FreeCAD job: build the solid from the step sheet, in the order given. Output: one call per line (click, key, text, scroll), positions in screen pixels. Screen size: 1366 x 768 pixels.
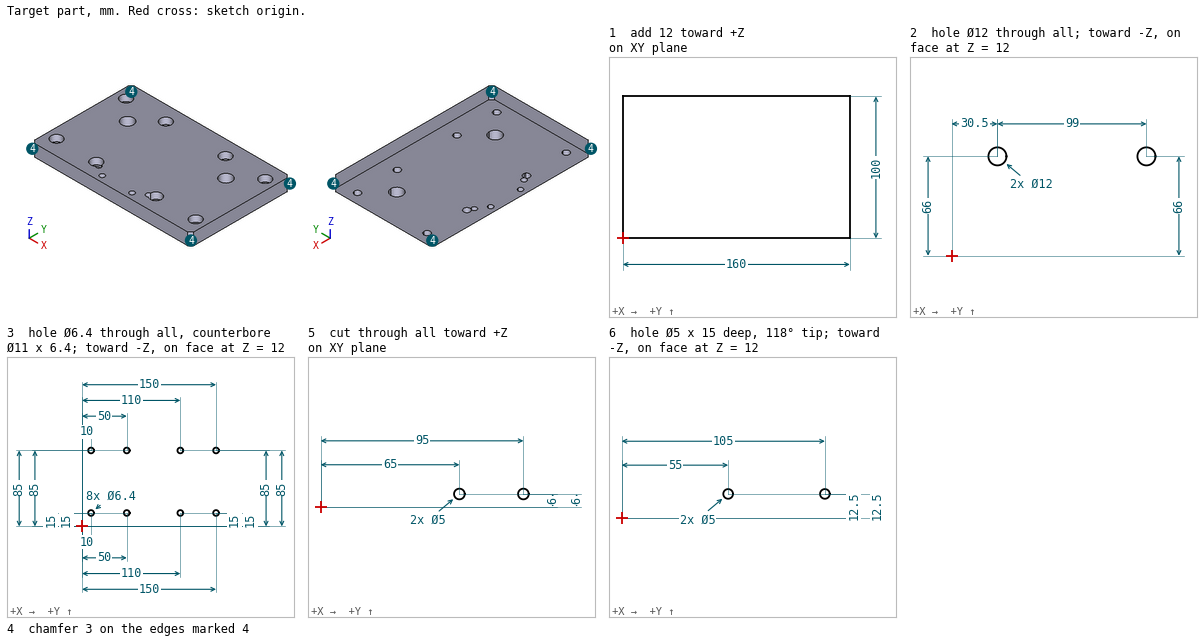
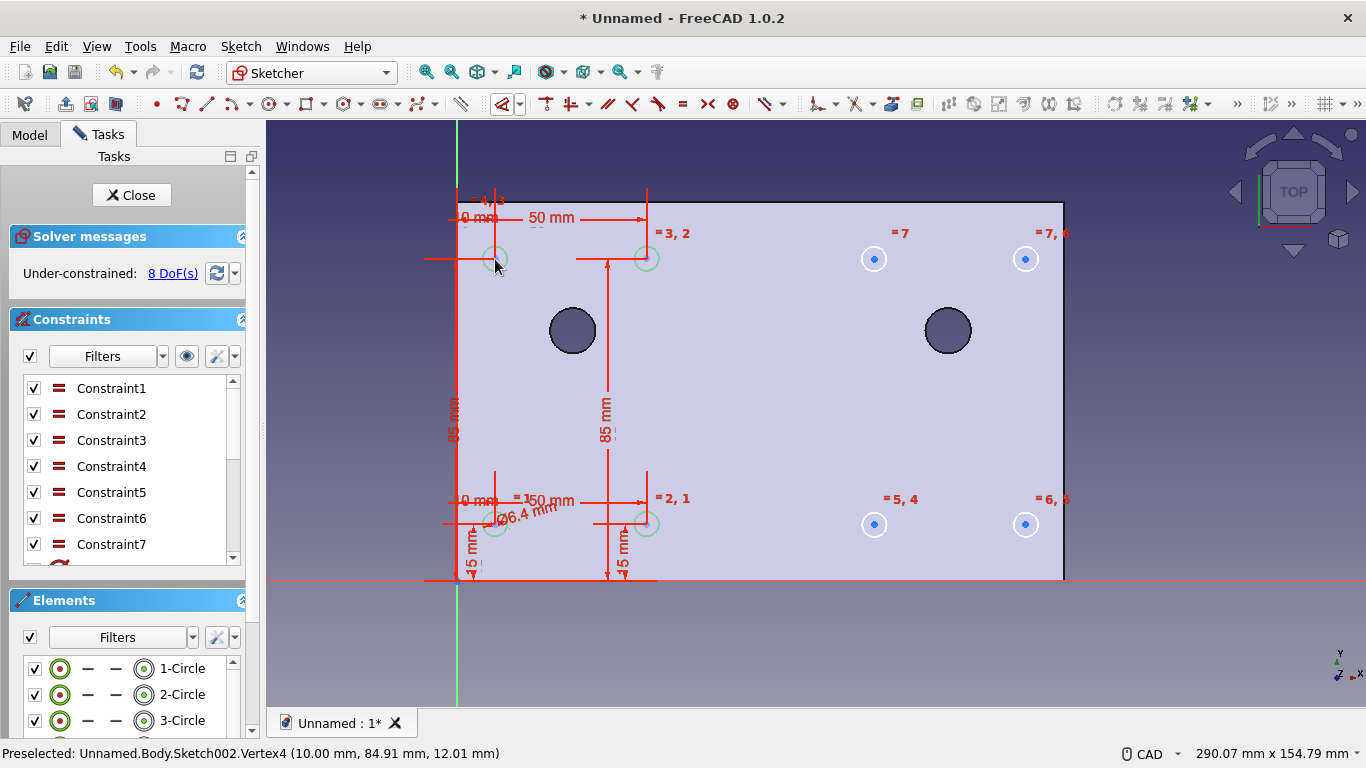
click(874, 525)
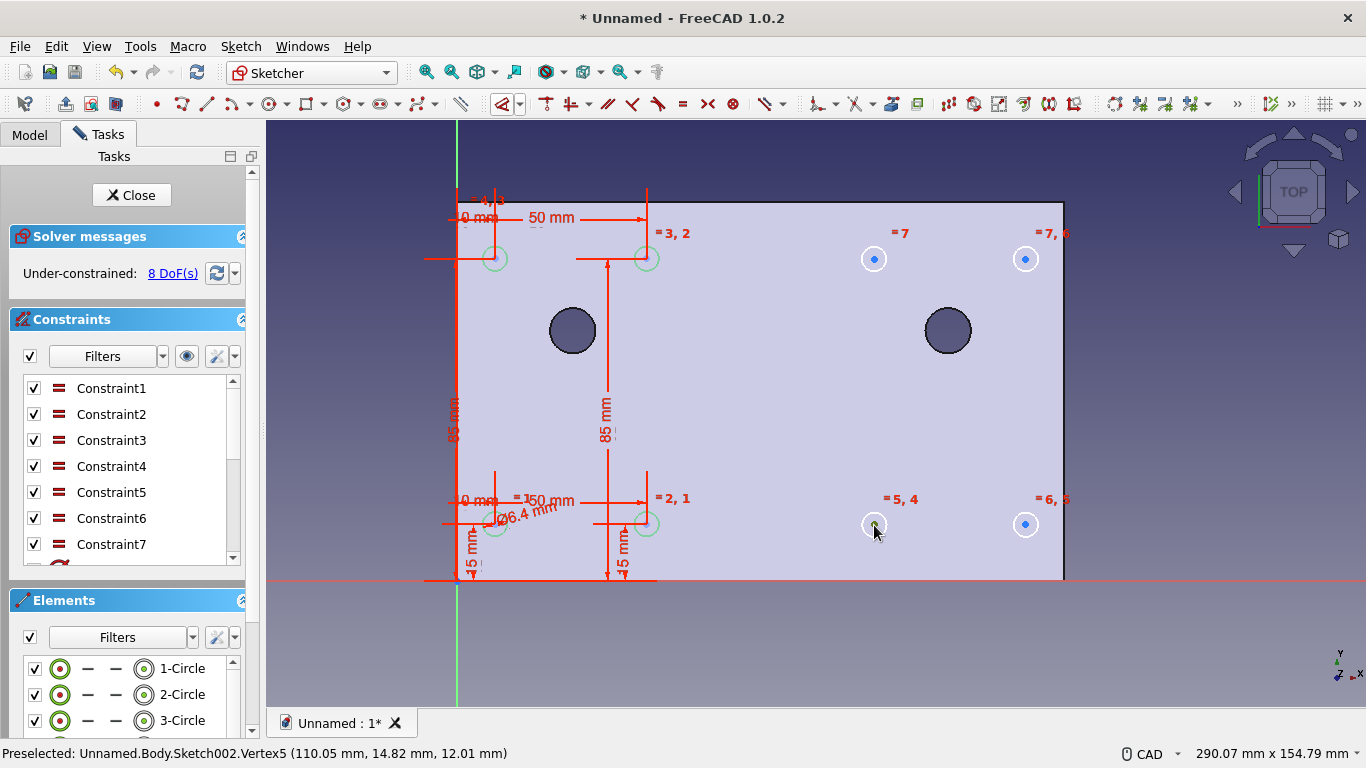
click(520, 104)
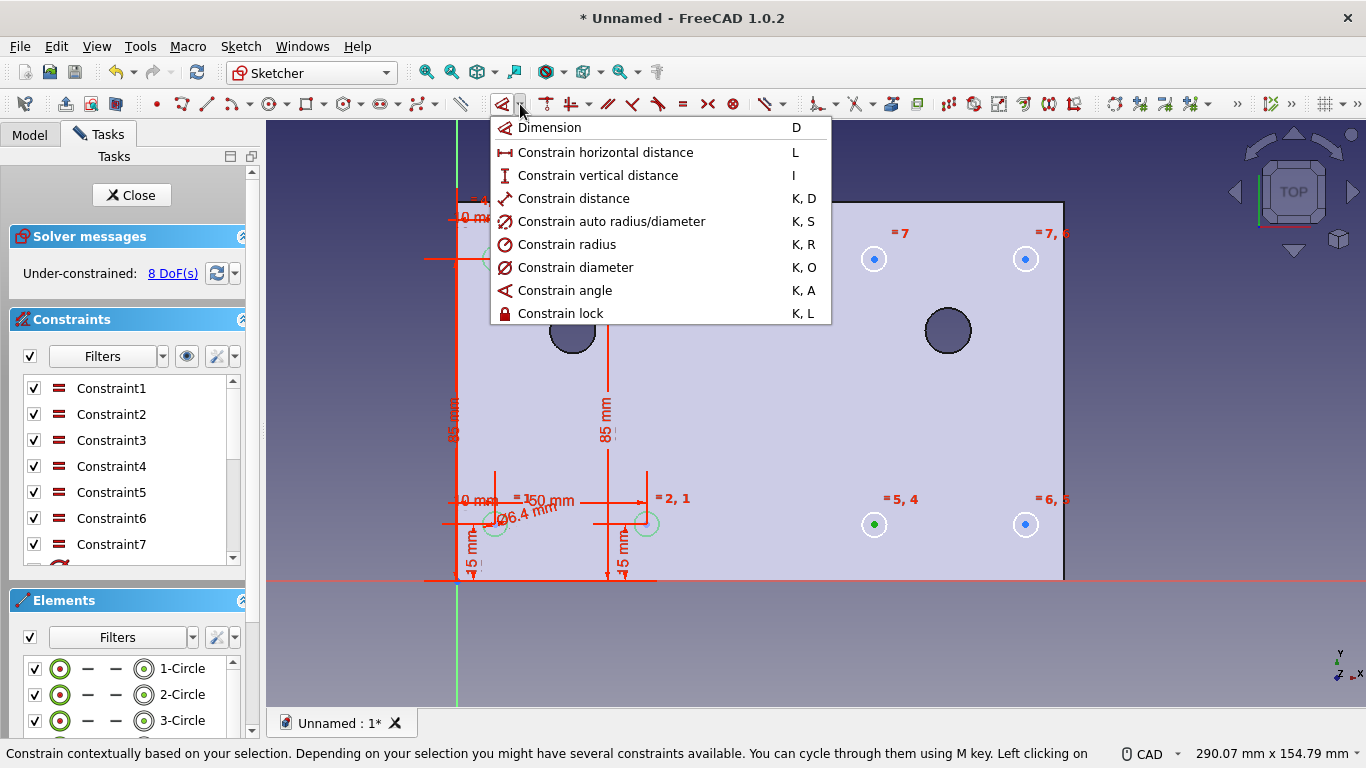
click(661, 176)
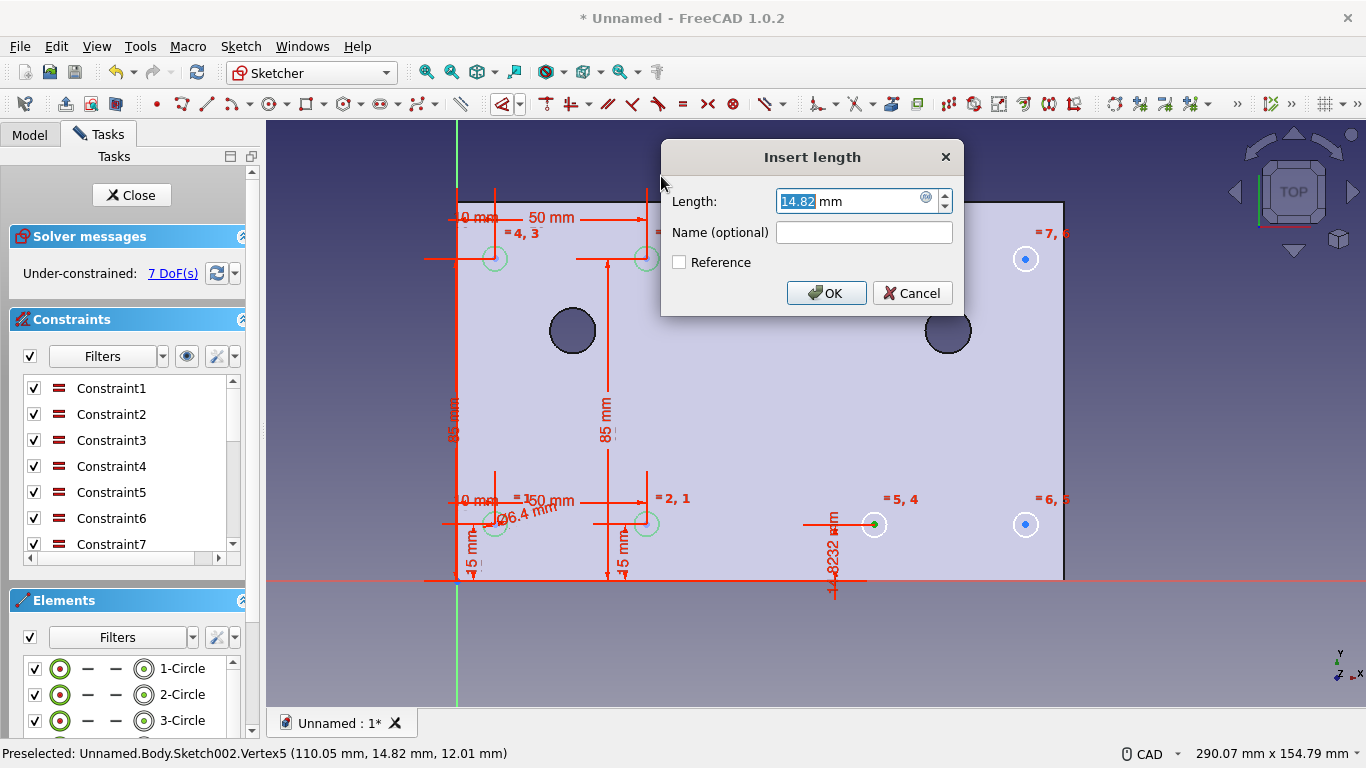
text(15)
key(Return)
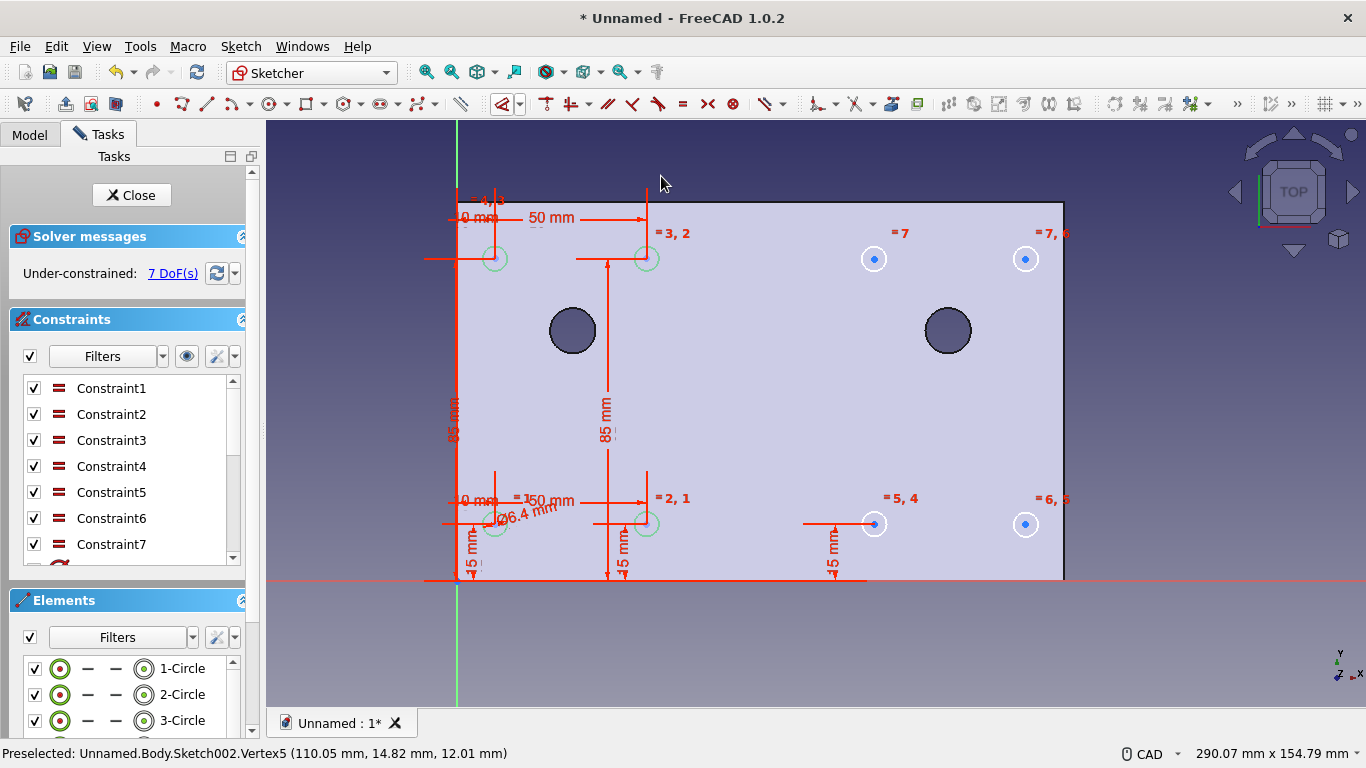
click(1026, 525)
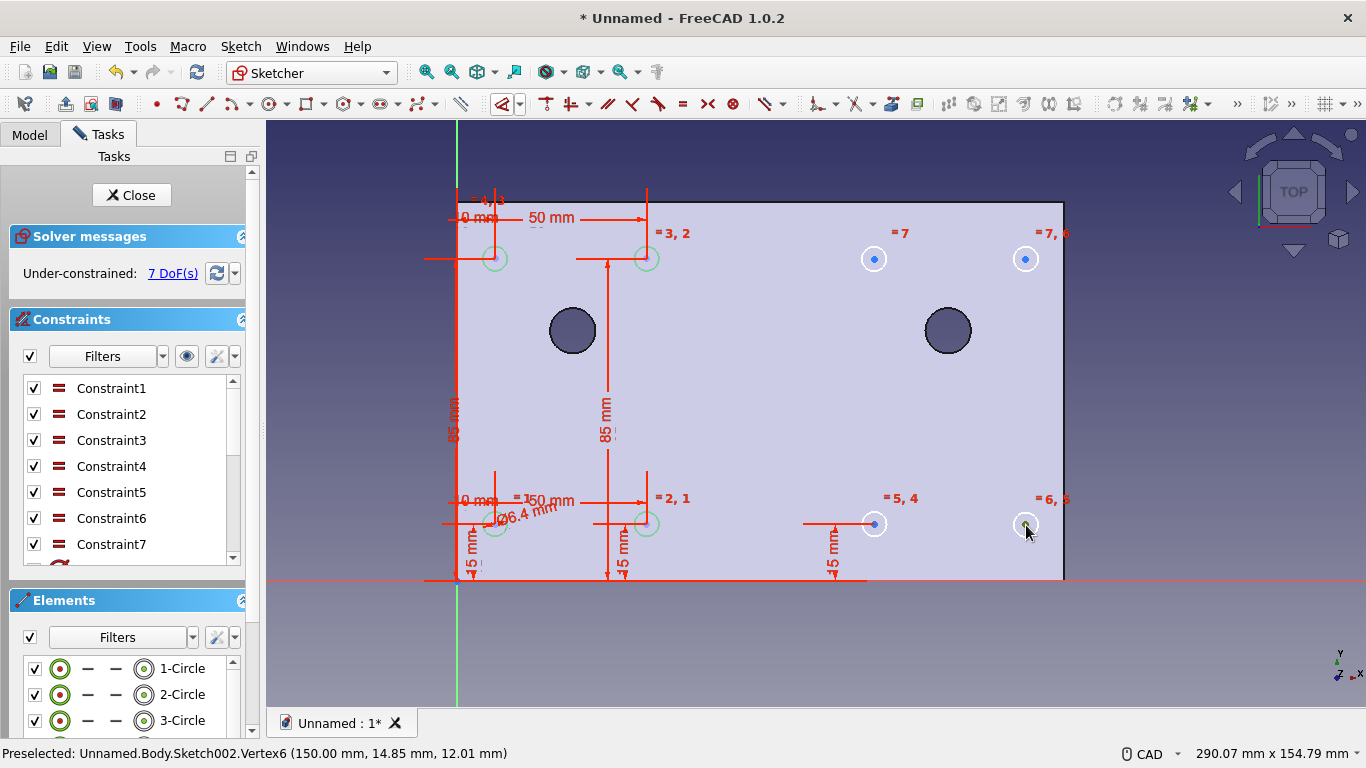
click(520, 104)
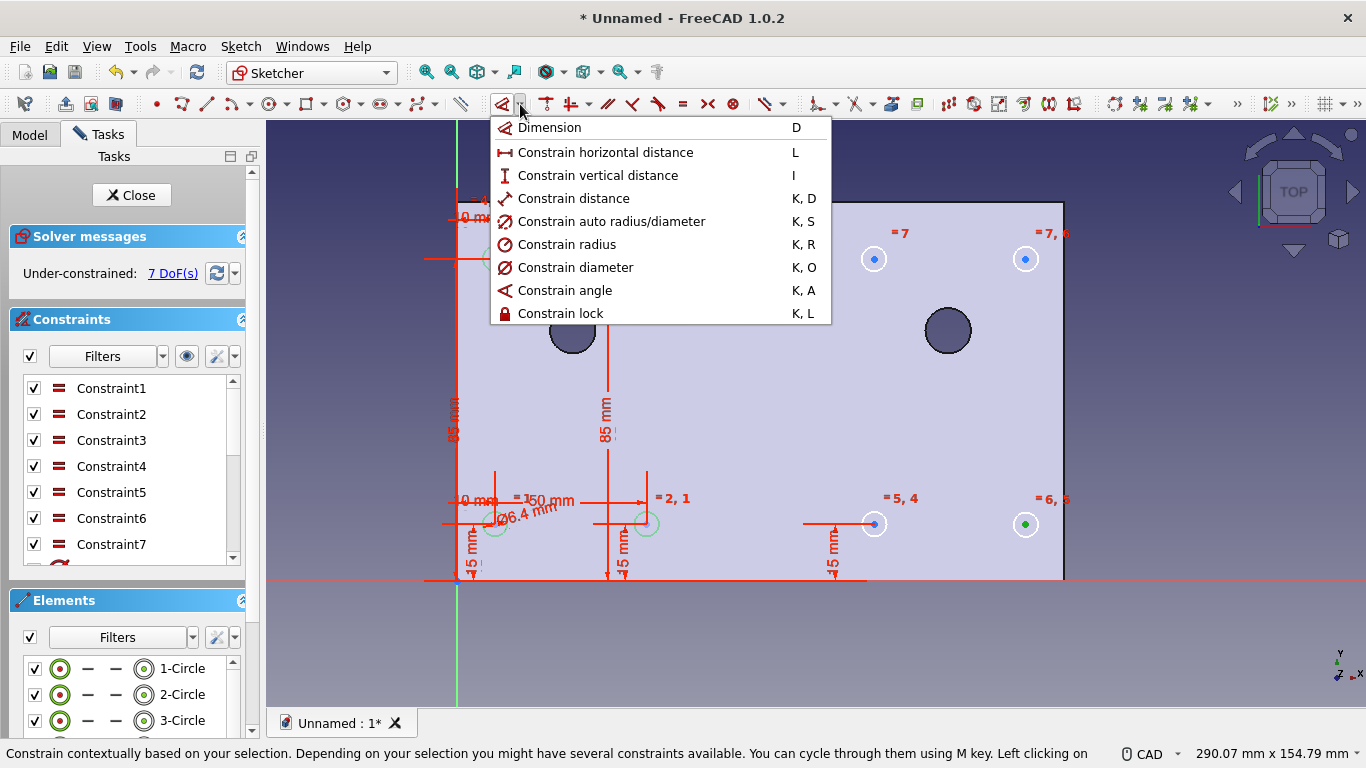
click(661, 176)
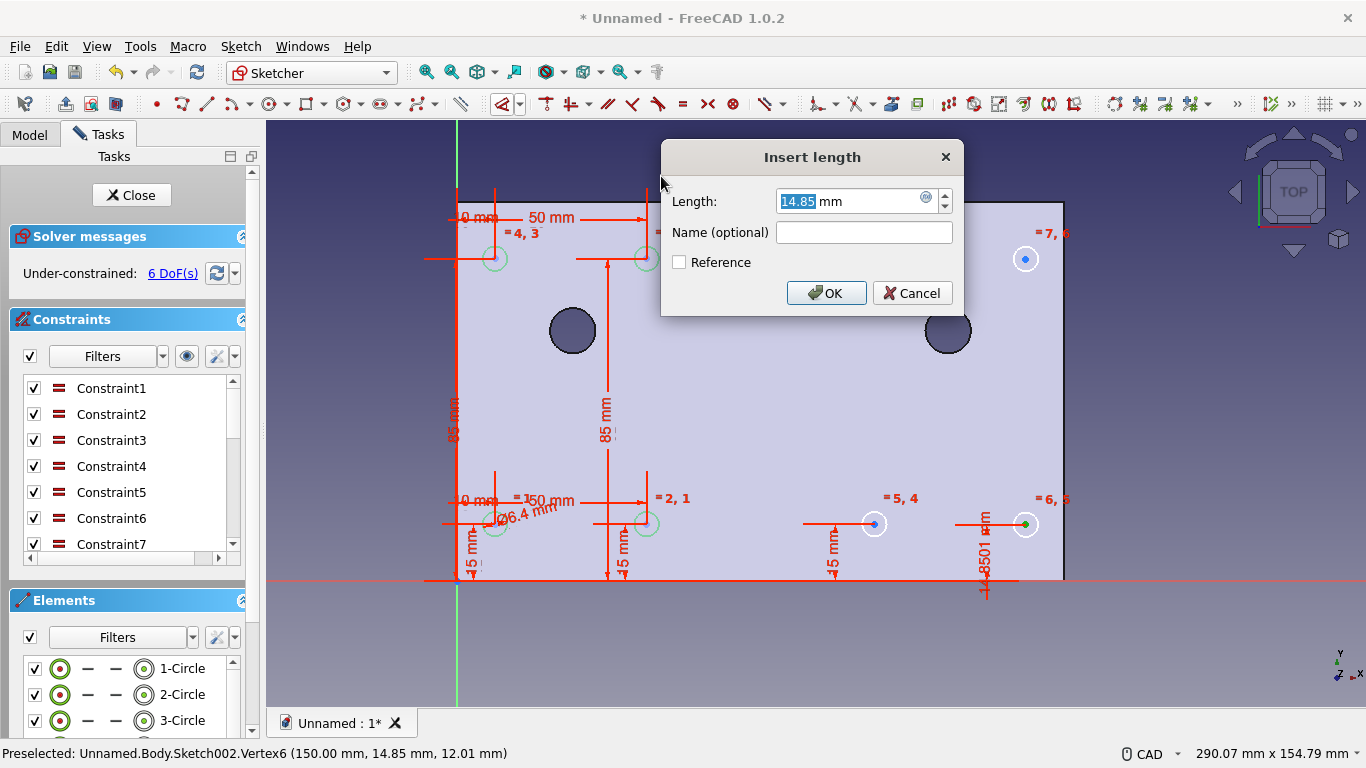
text(15)
key(Return)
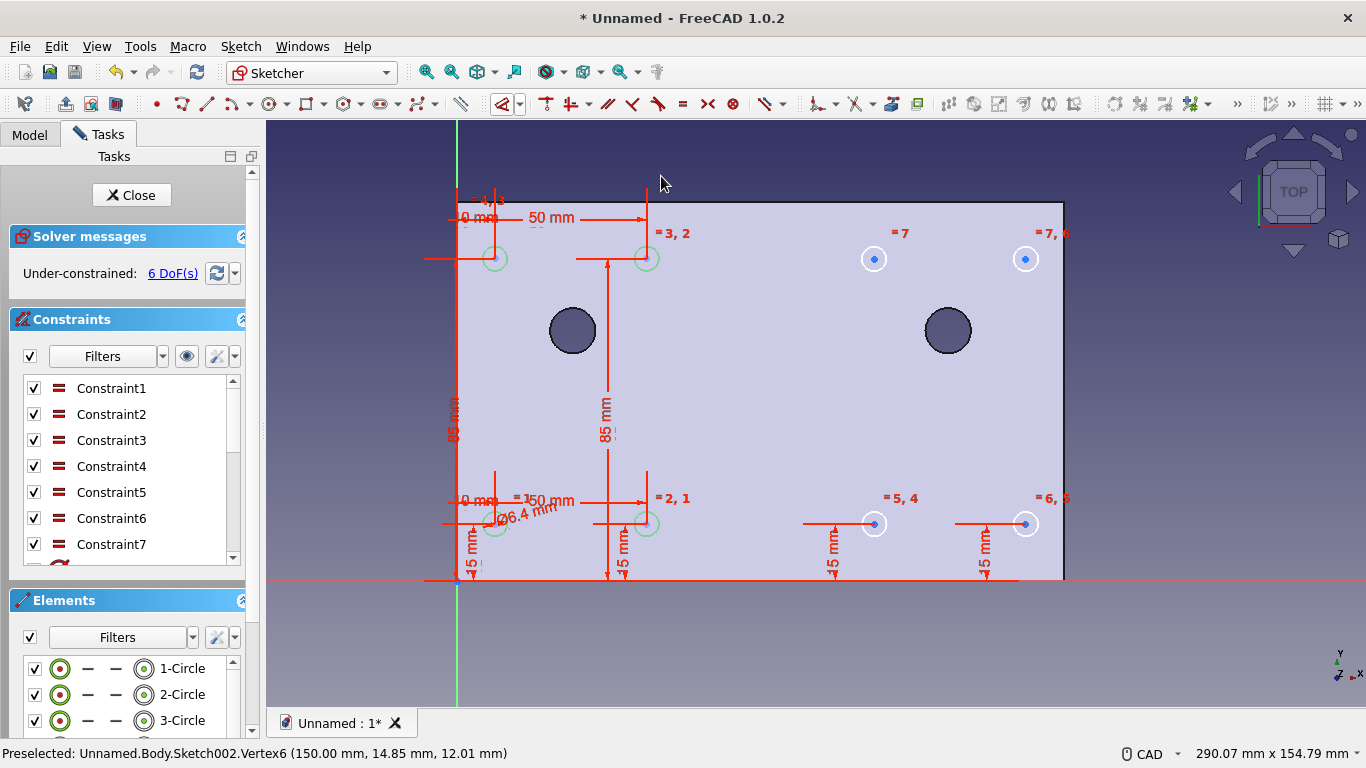
click(1026, 259)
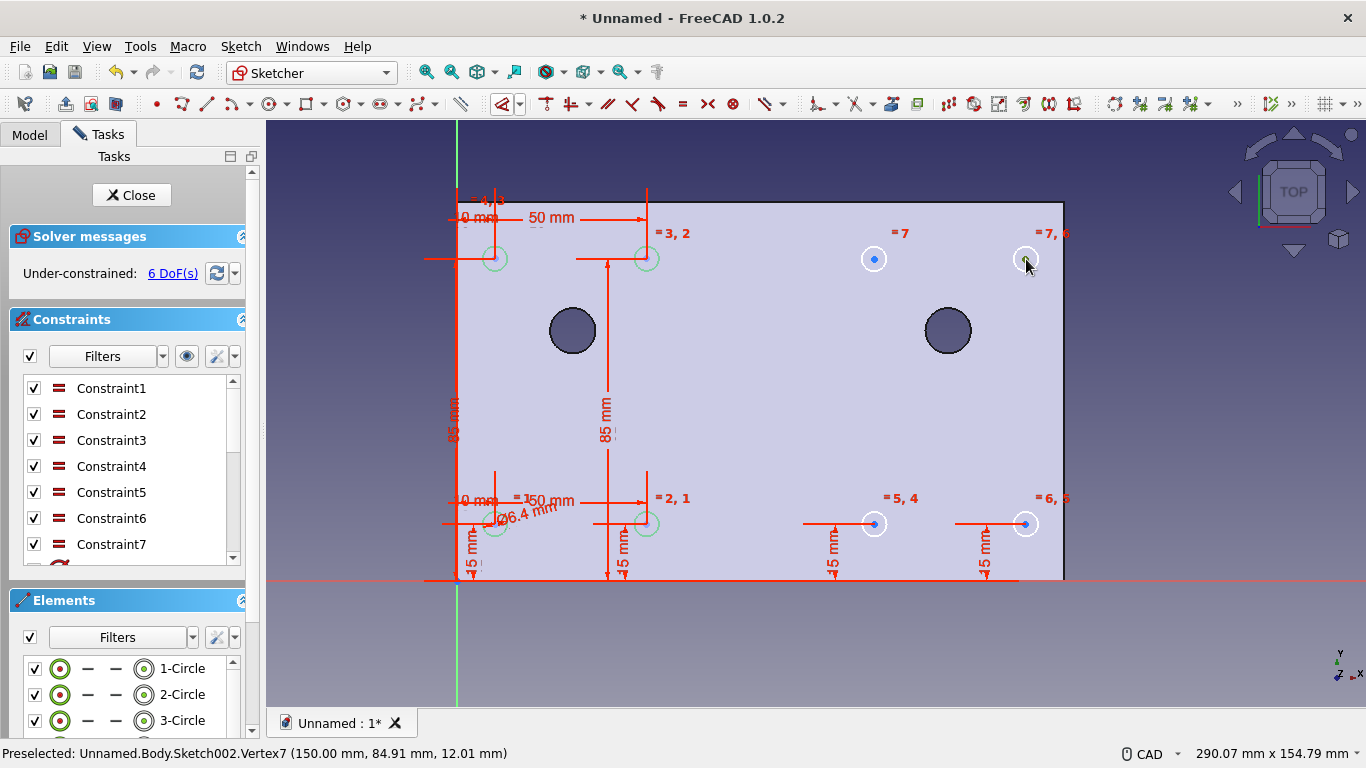
key(i)